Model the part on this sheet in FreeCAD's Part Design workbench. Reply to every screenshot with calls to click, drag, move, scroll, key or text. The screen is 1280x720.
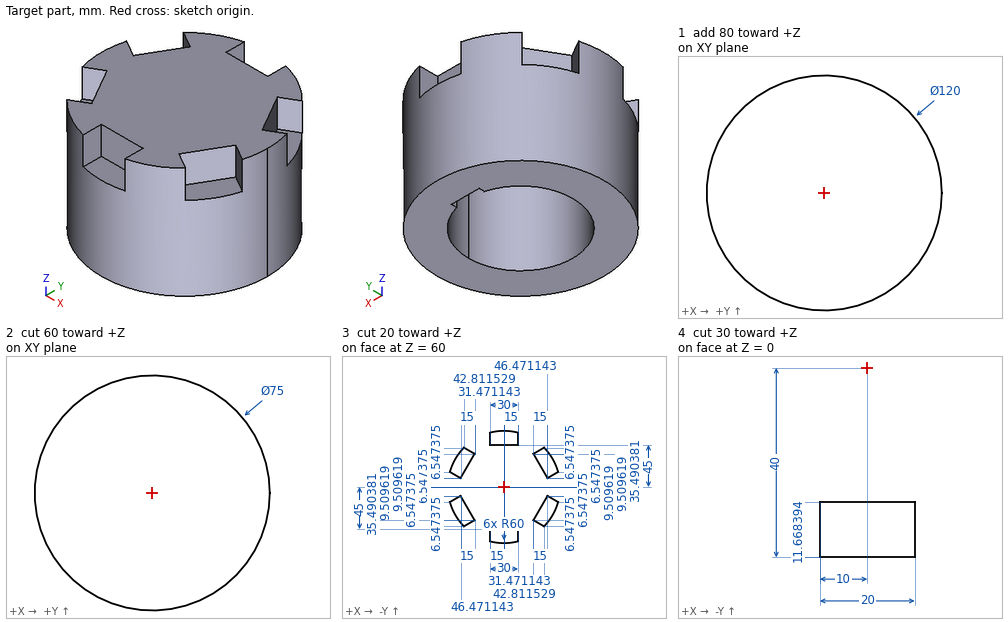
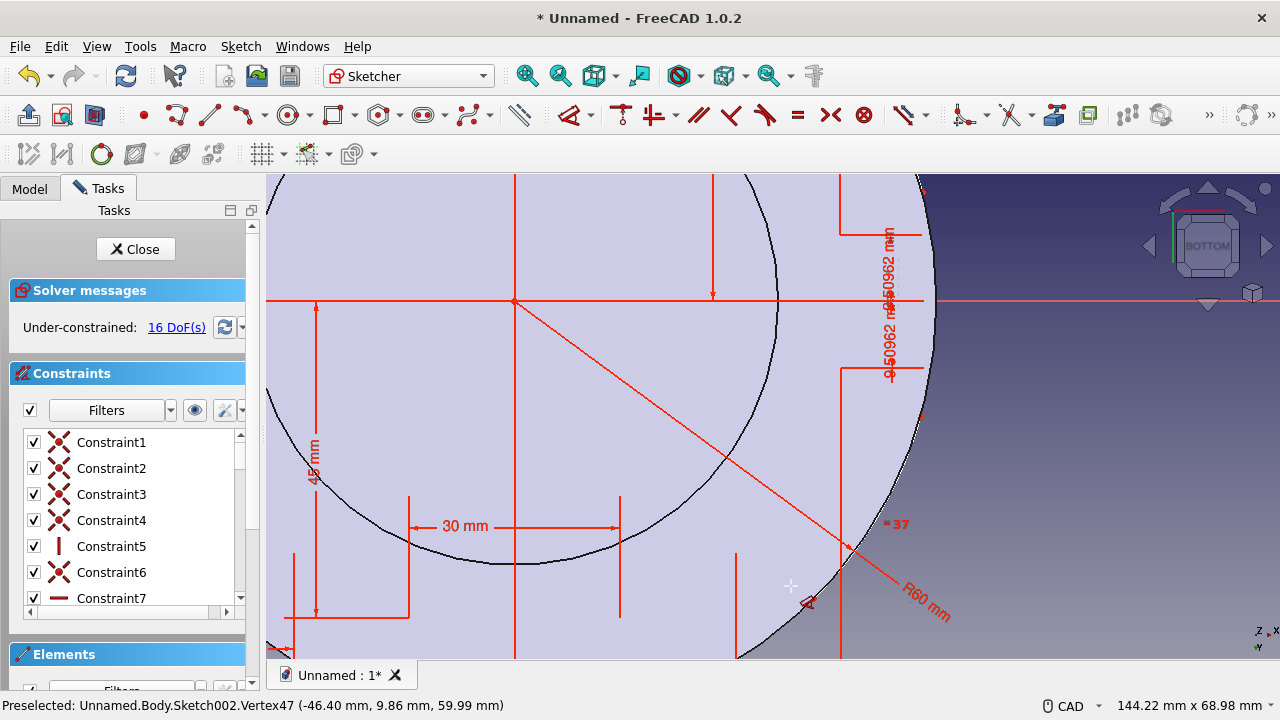
click(790, 585)
click(848, 587)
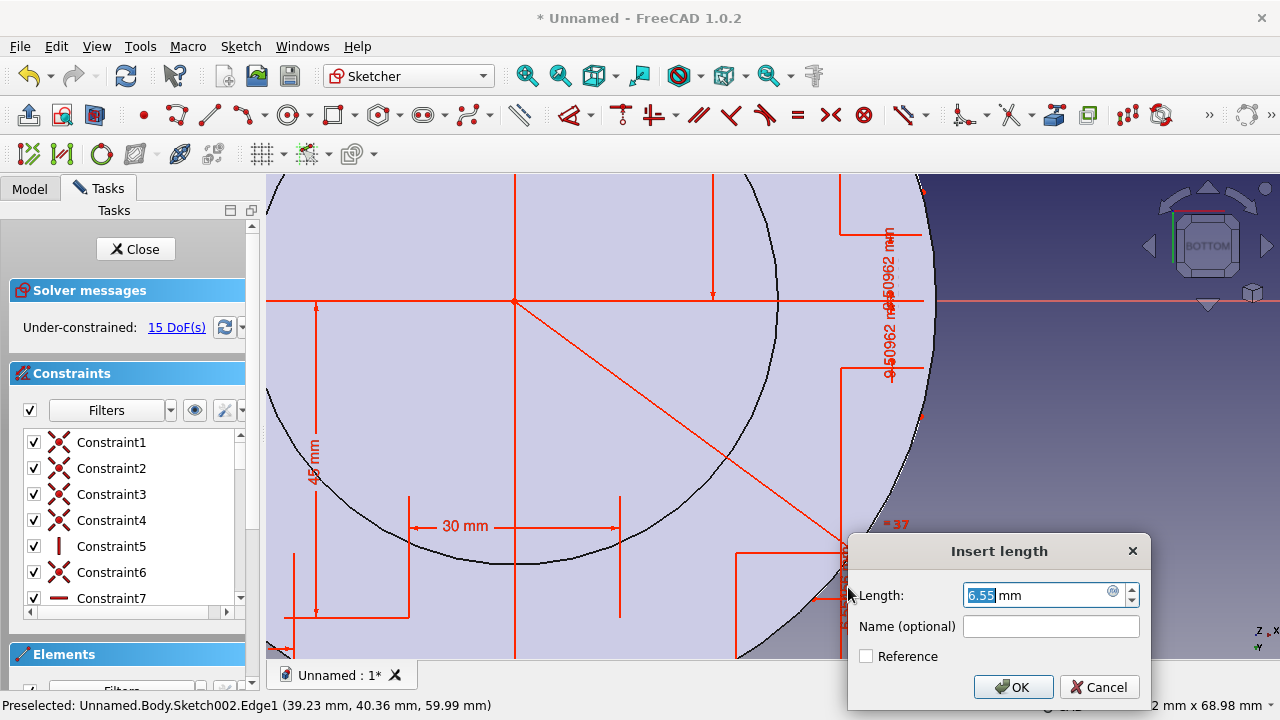
text(6.547375)
key(Return)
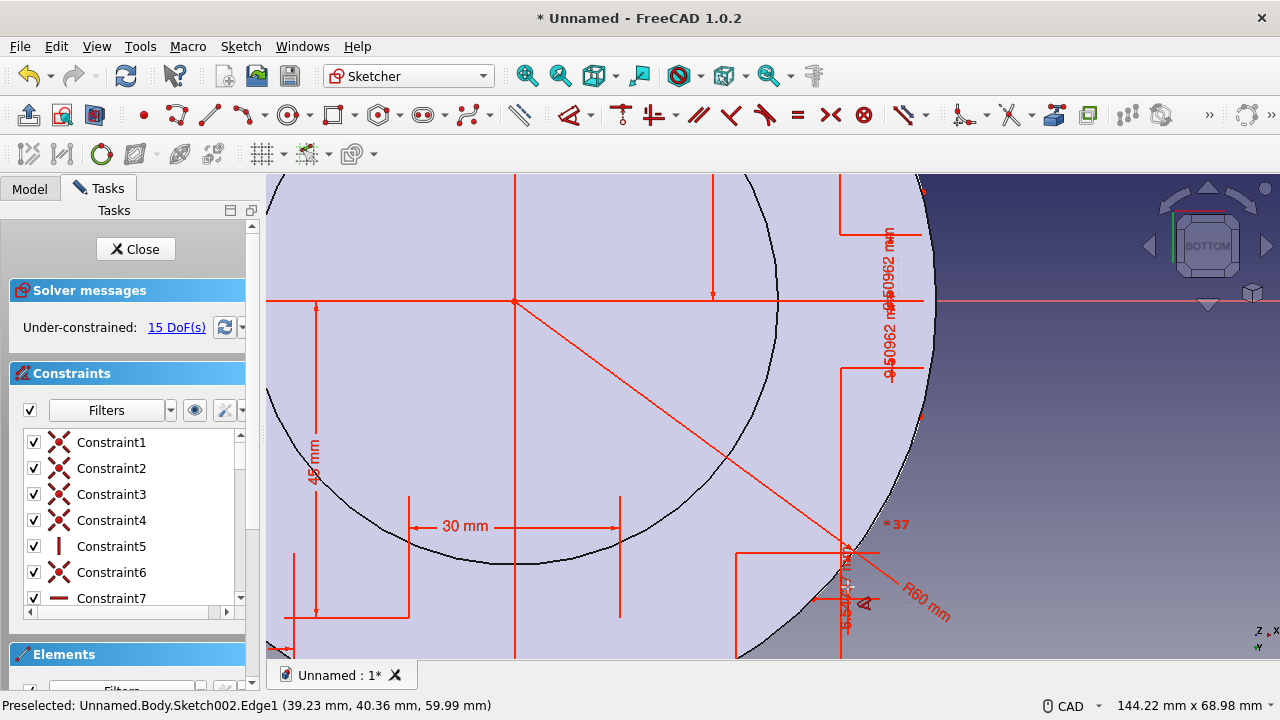
click(865, 383)
click(954, 393)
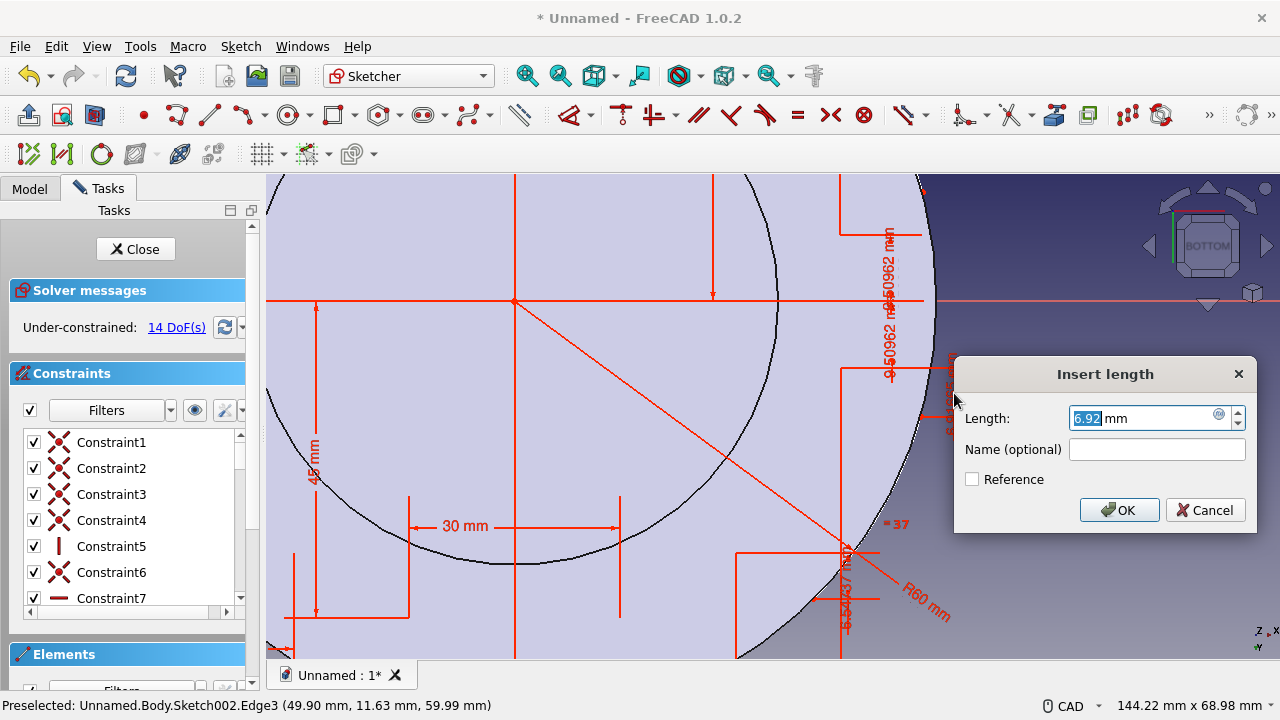
text(6.547375)
key(Return)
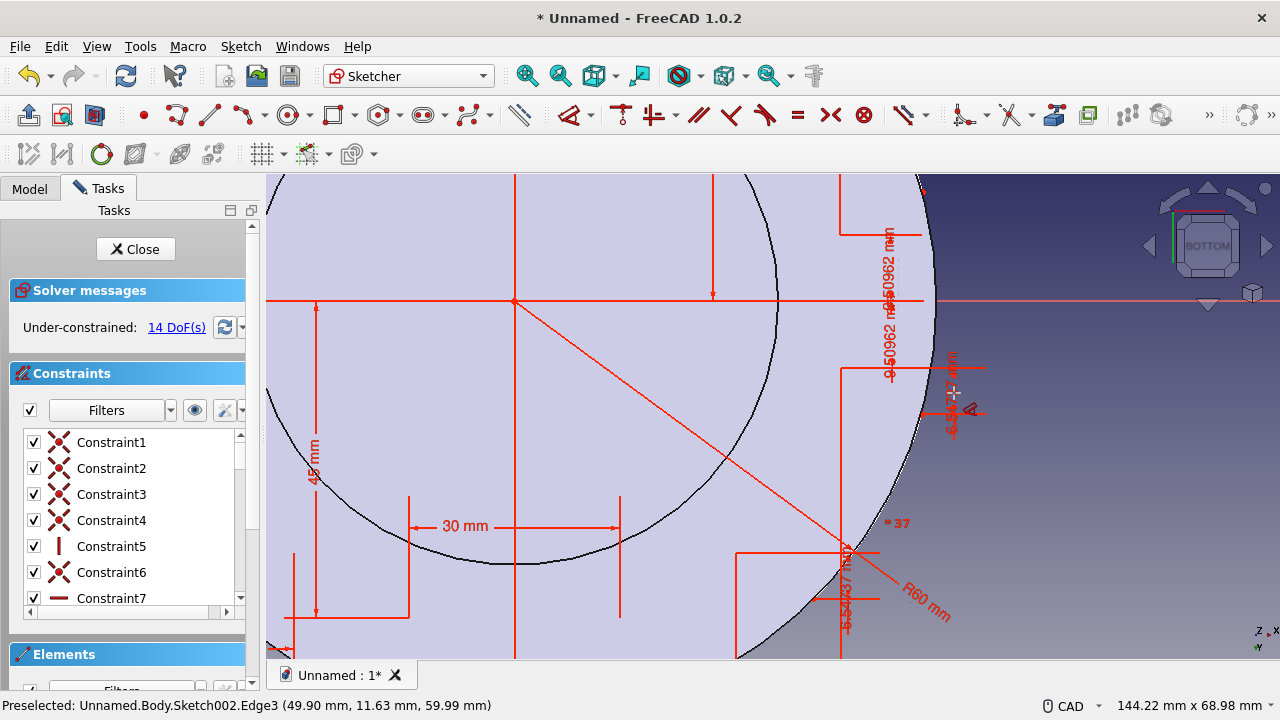
click(898, 205)
click(956, 218)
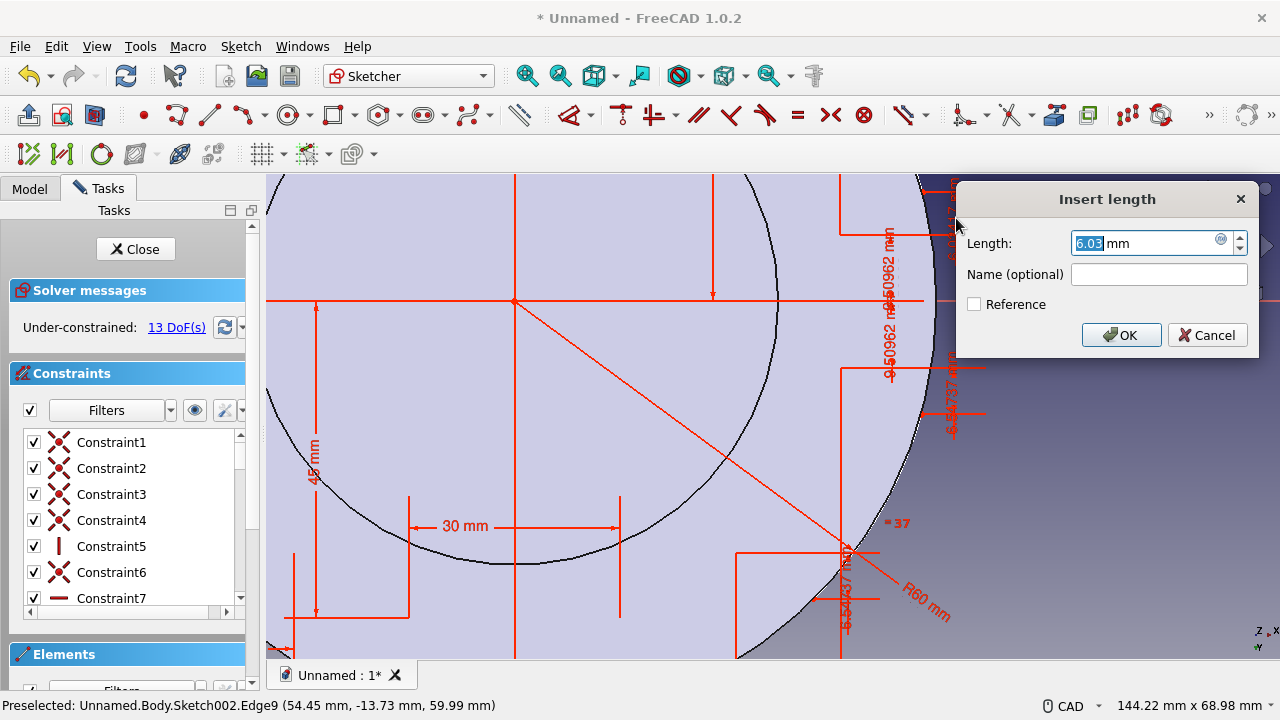
text(6.547375)
key(Return)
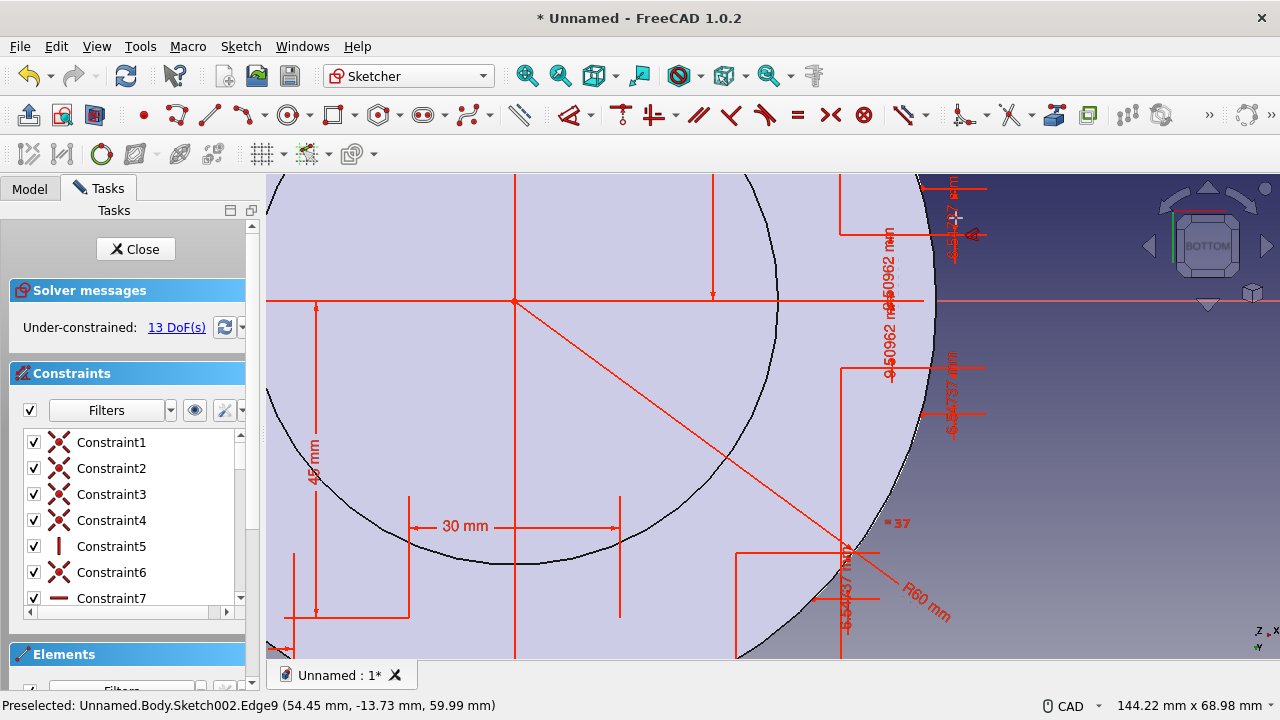
scroll(815, 483, down, 5)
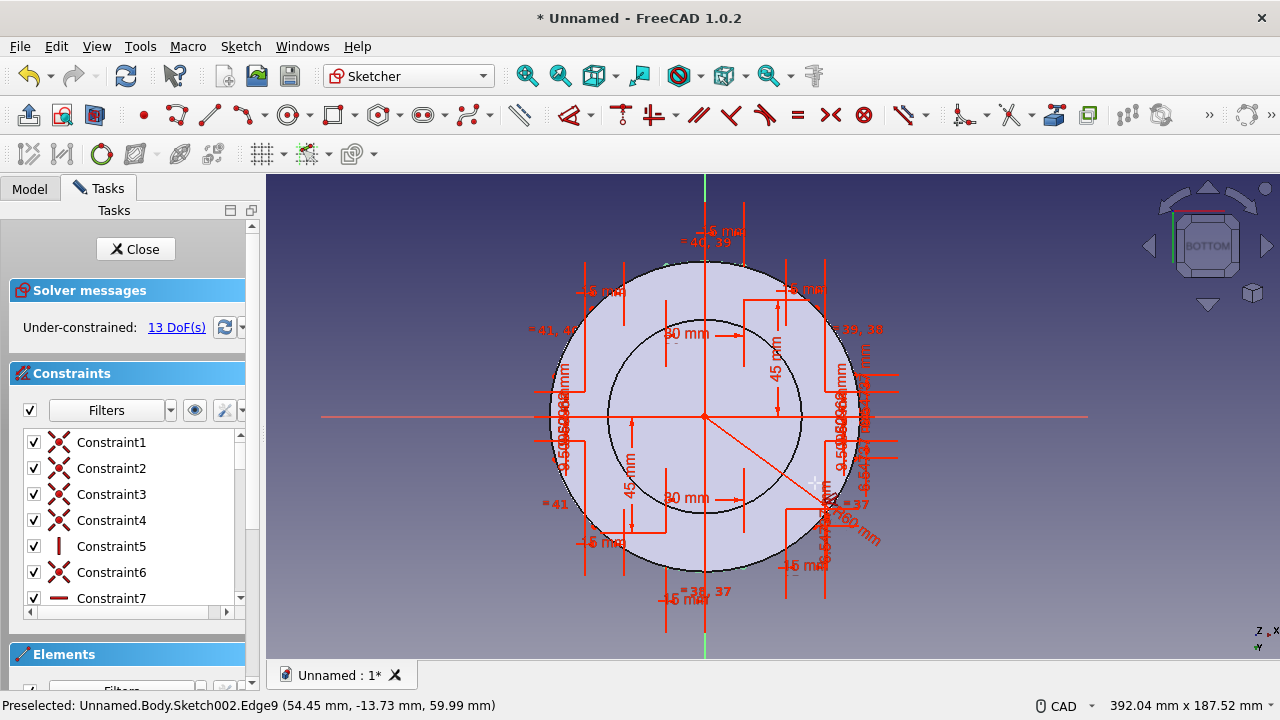
scroll(795, 320, up, 5)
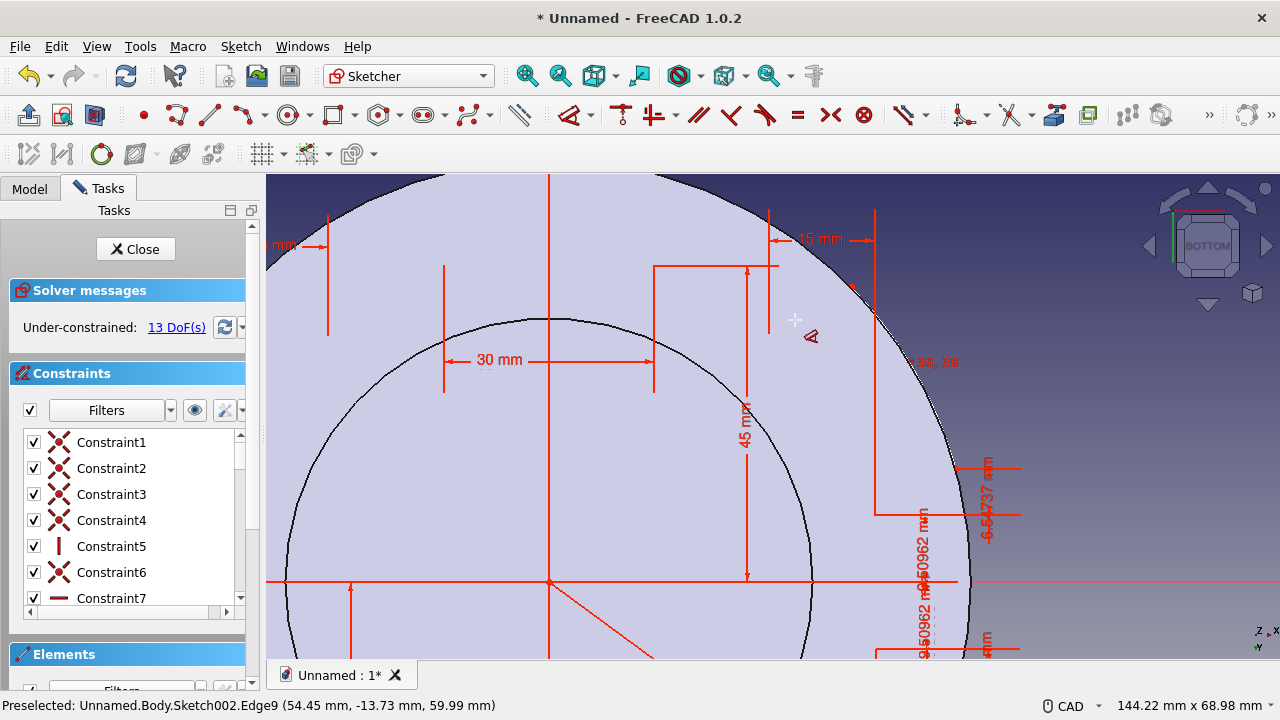
click(794, 320)
click(885, 300)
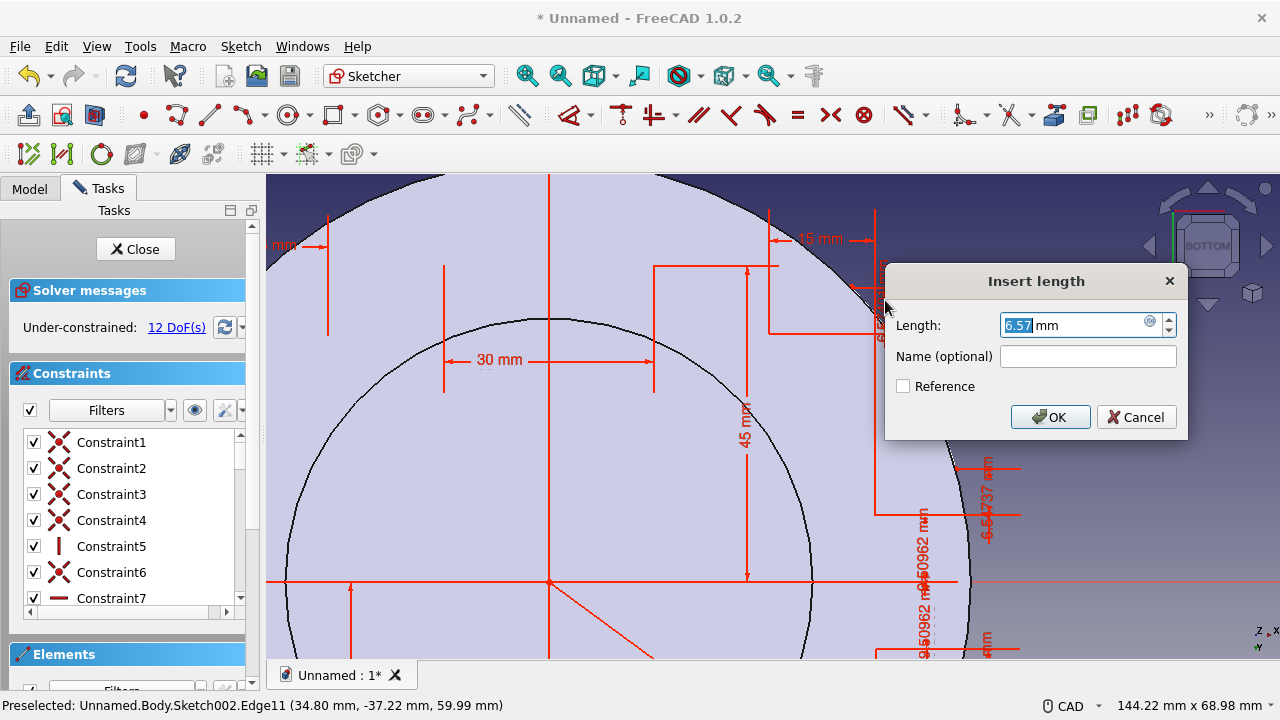
text(6.547375)
key(Return)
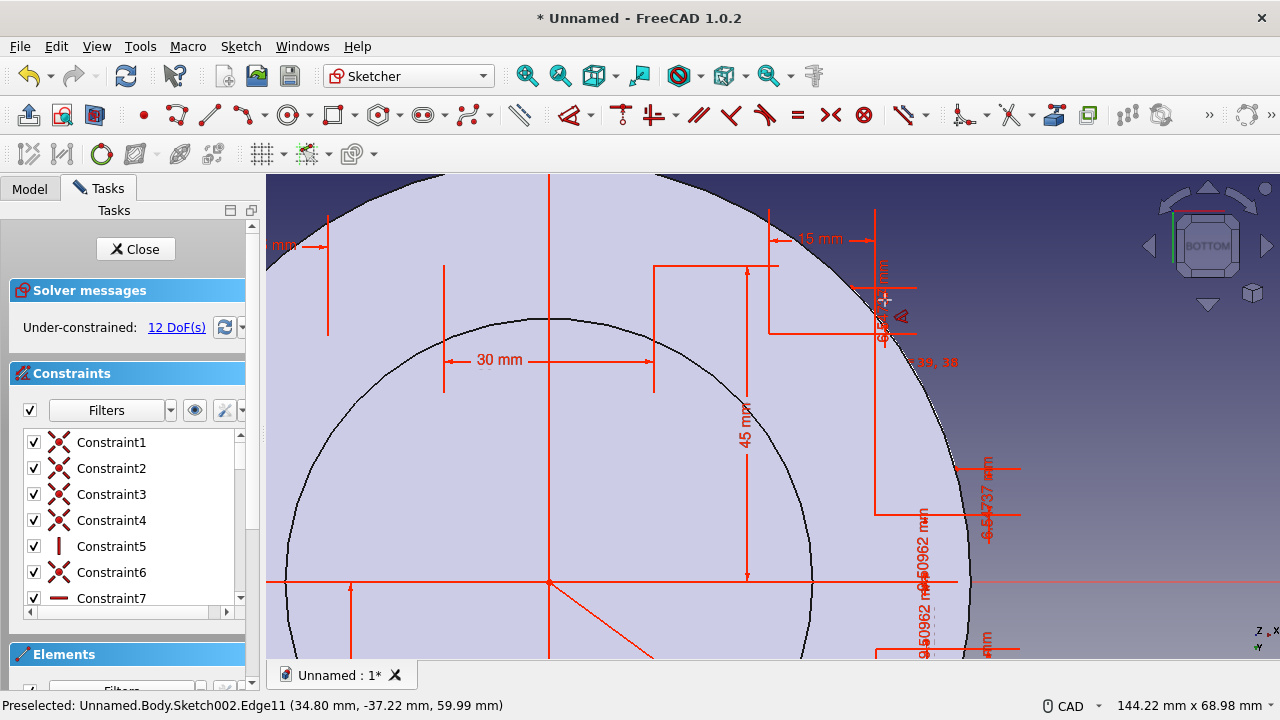
click(303, 322)
click(362, 313)